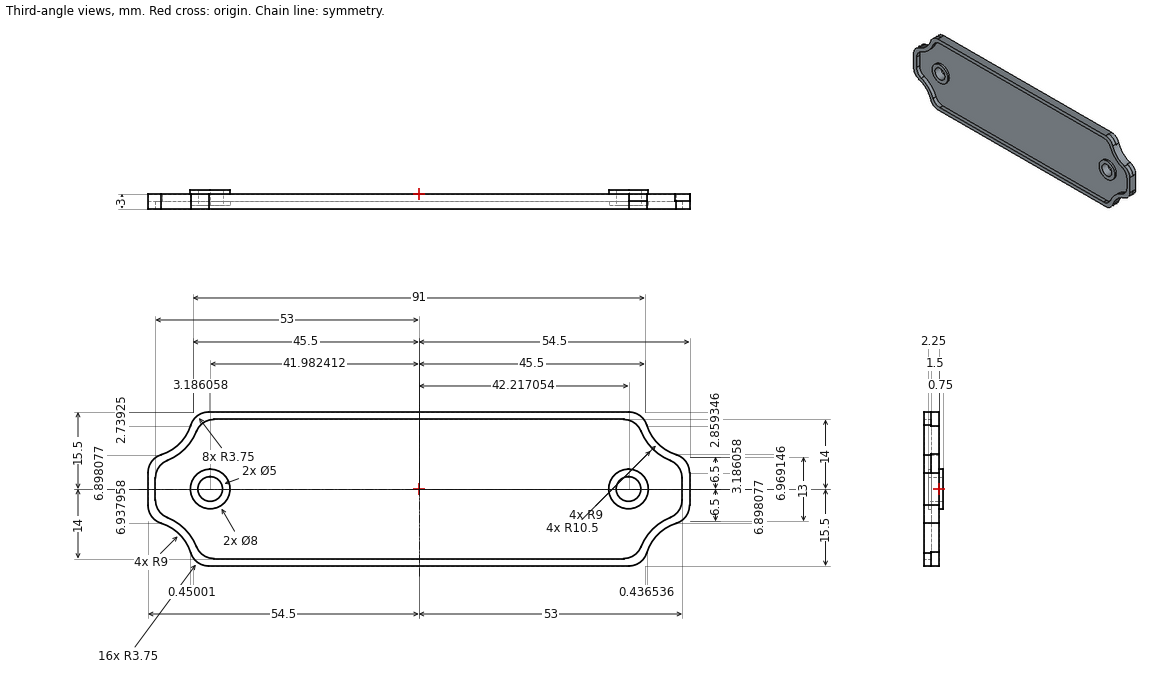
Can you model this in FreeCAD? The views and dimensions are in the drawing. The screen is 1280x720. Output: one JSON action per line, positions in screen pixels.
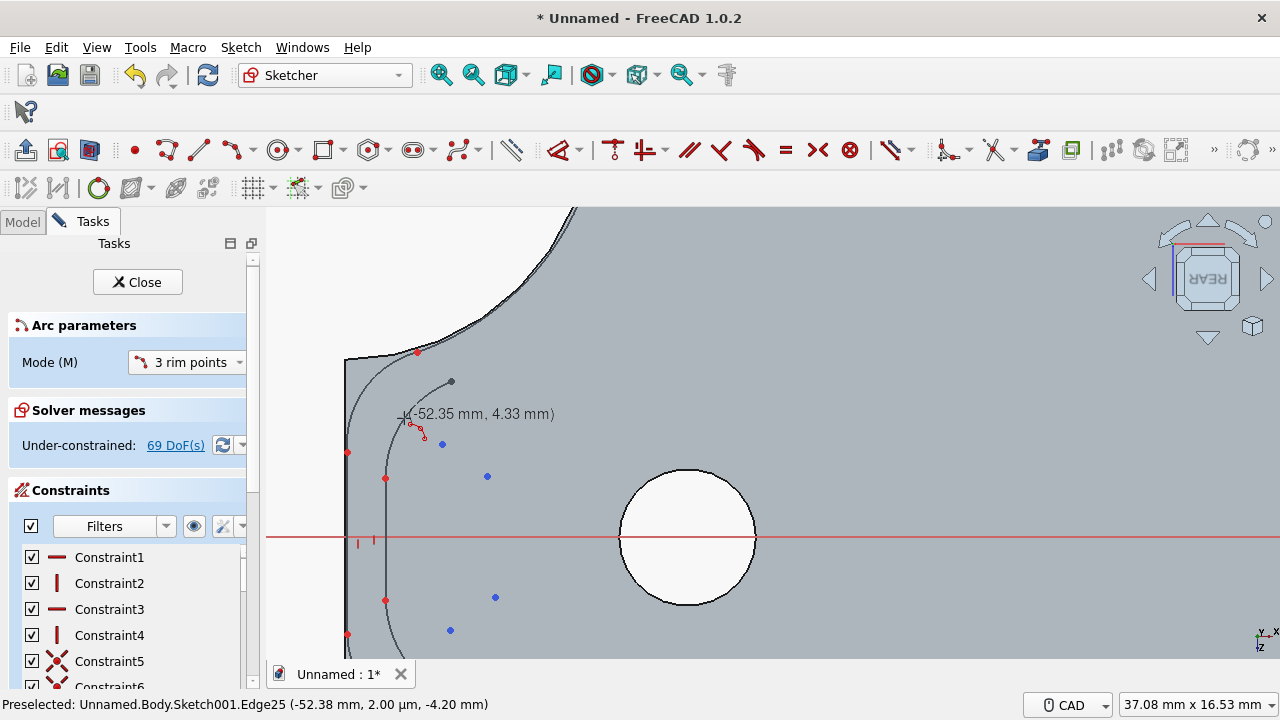
{"action": "left_click", "coordinate": [452, 382]}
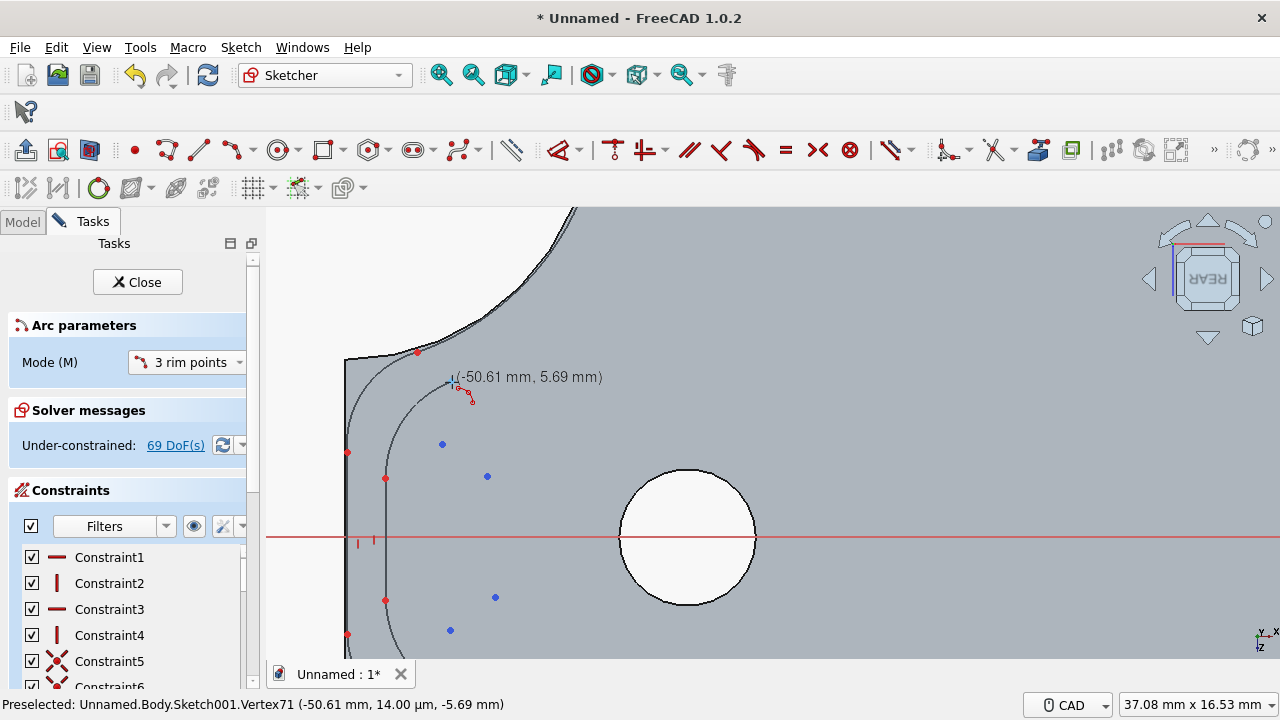
{"action": "scroll", "coordinate": [418, 407], "scroll_direction": "down", "scroll_amount": 8}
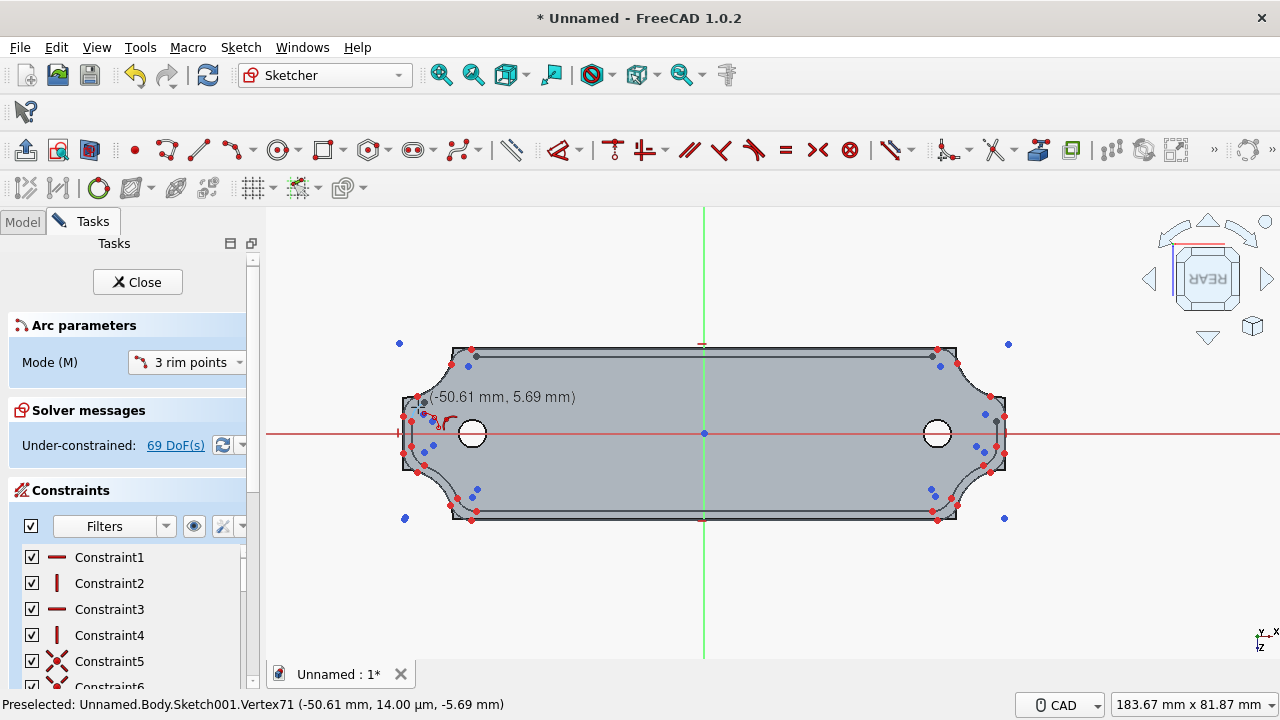
{"action": "scroll", "coordinate": [457, 369], "scroll_direction": "up", "scroll_amount": 4}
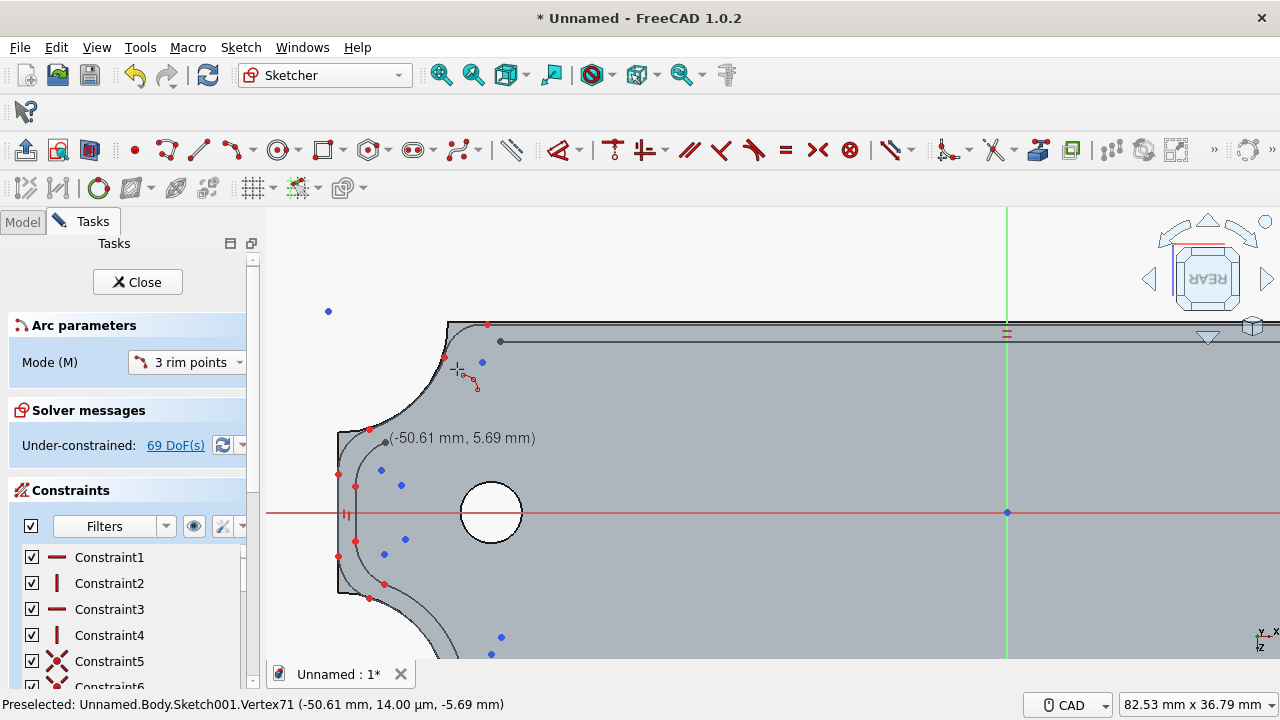
{"action": "left_click", "coordinate": [457, 370]}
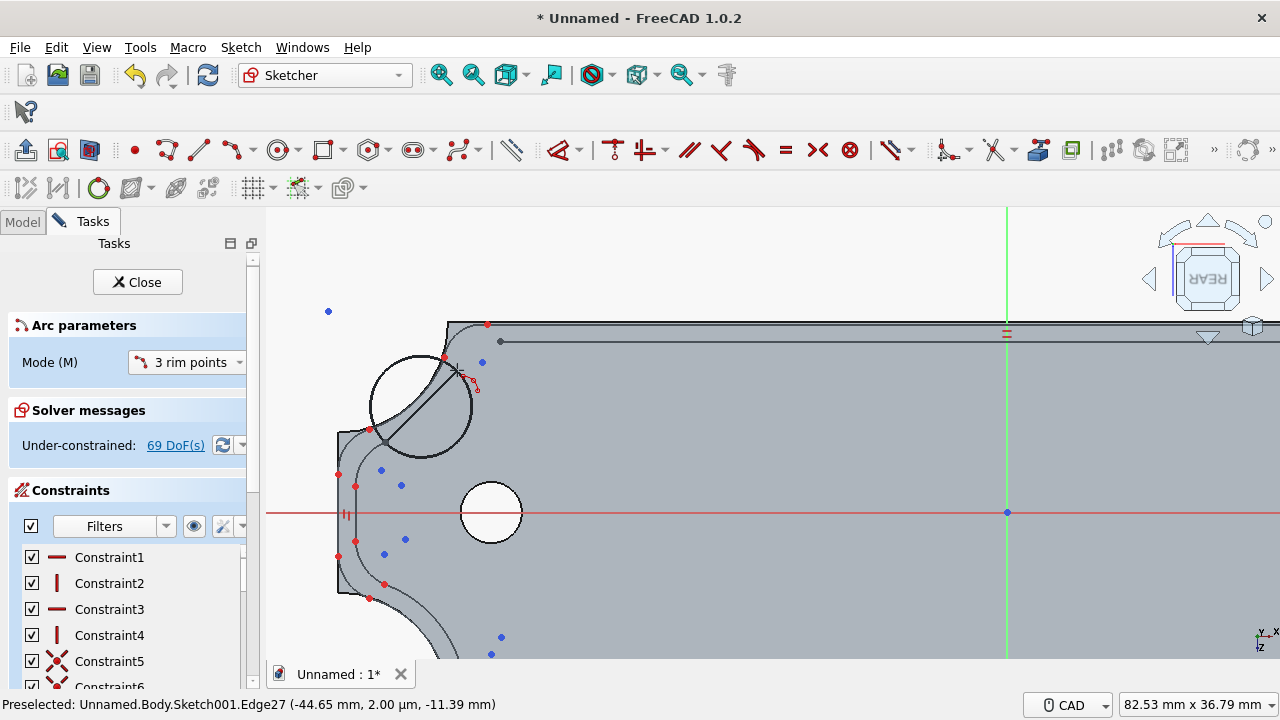
{"action": "scroll", "coordinate": [429, 413], "scroll_direction": "up", "scroll_amount": 3}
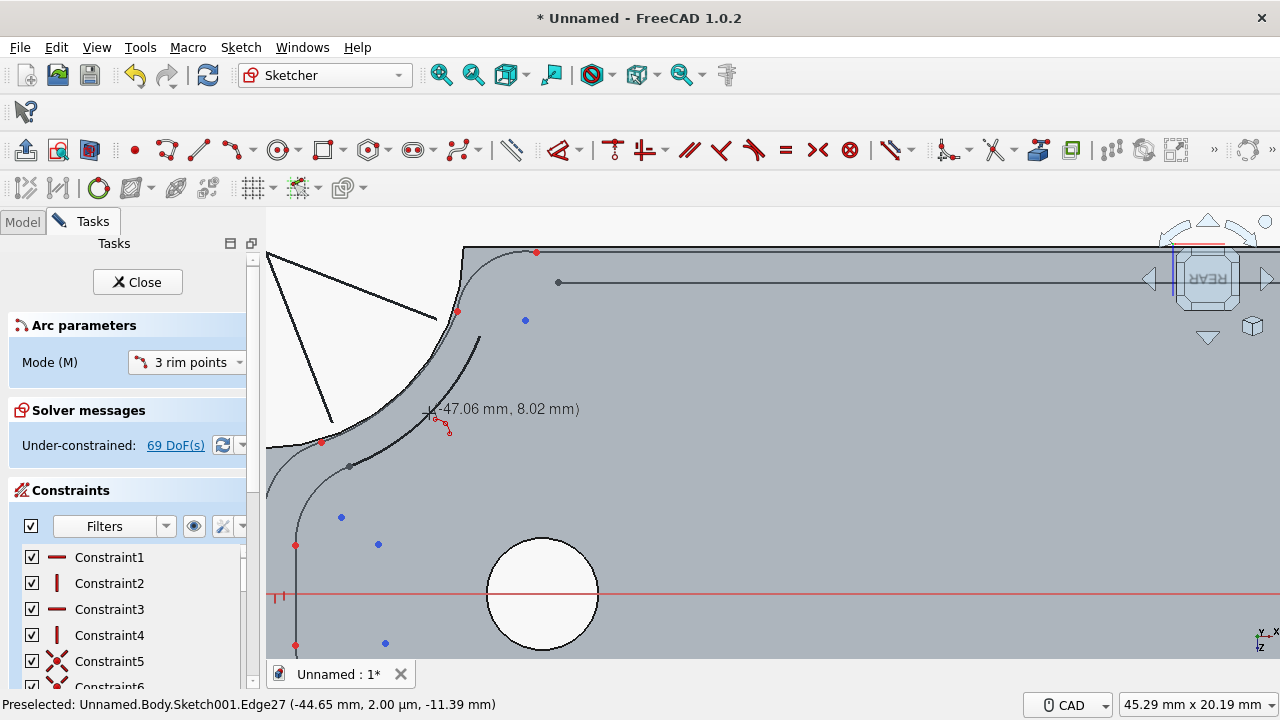
{"action": "left_click", "coordinate": [428, 413]}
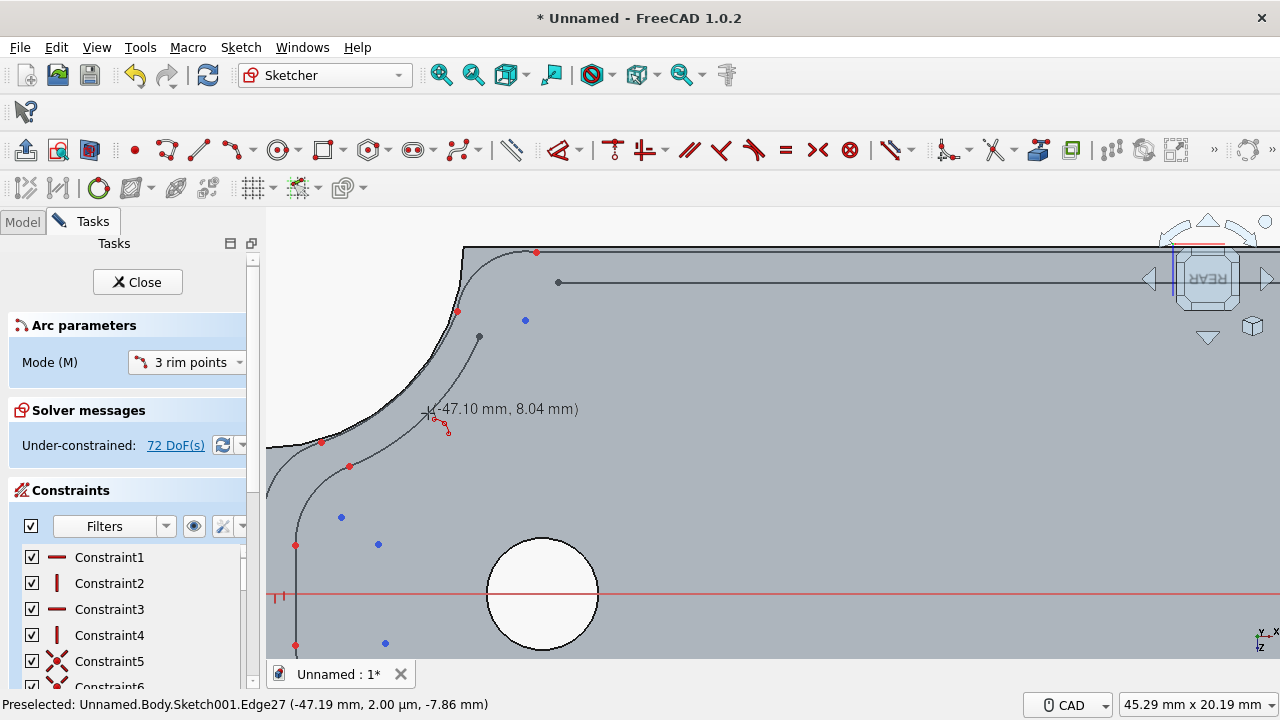
{"action": "left_click", "coordinate": [480, 336]}
{"action": "left_click", "coordinate": [558, 283]}
{"action": "left_click", "coordinate": [512, 295]}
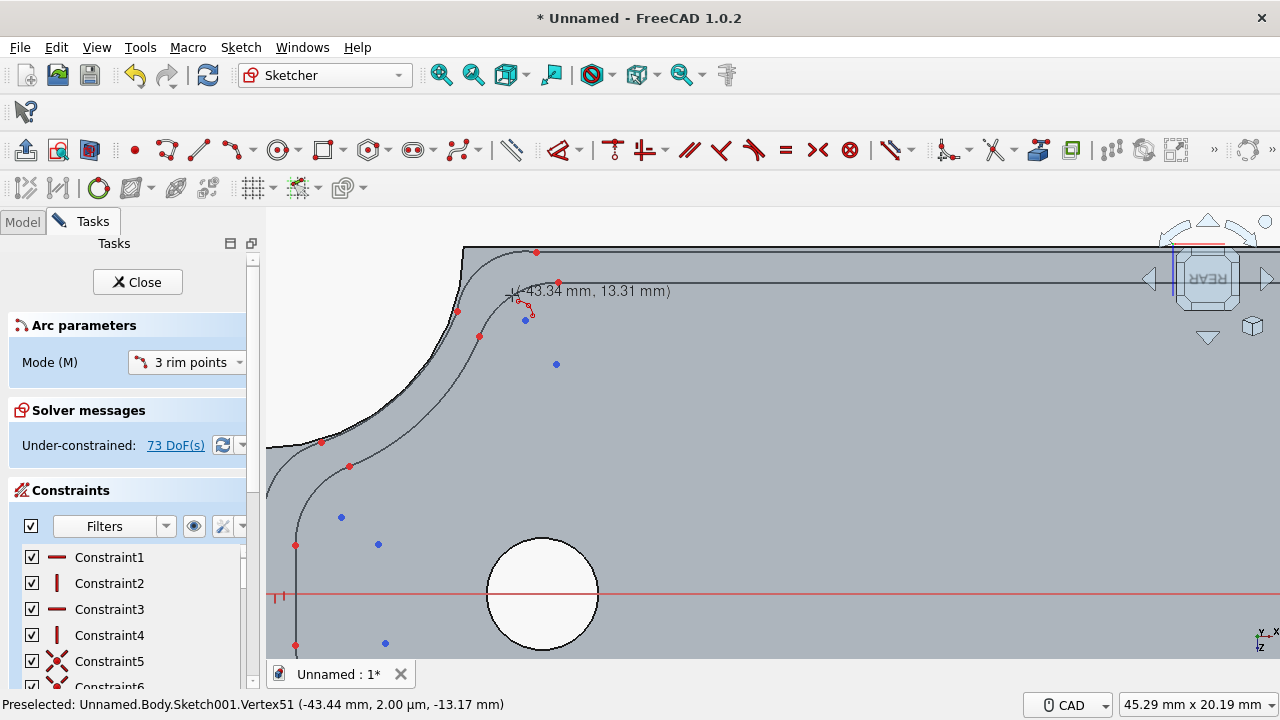
{"action": "scroll", "coordinate": [450, 380], "scroll_direction": "down", "scroll_amount": 7}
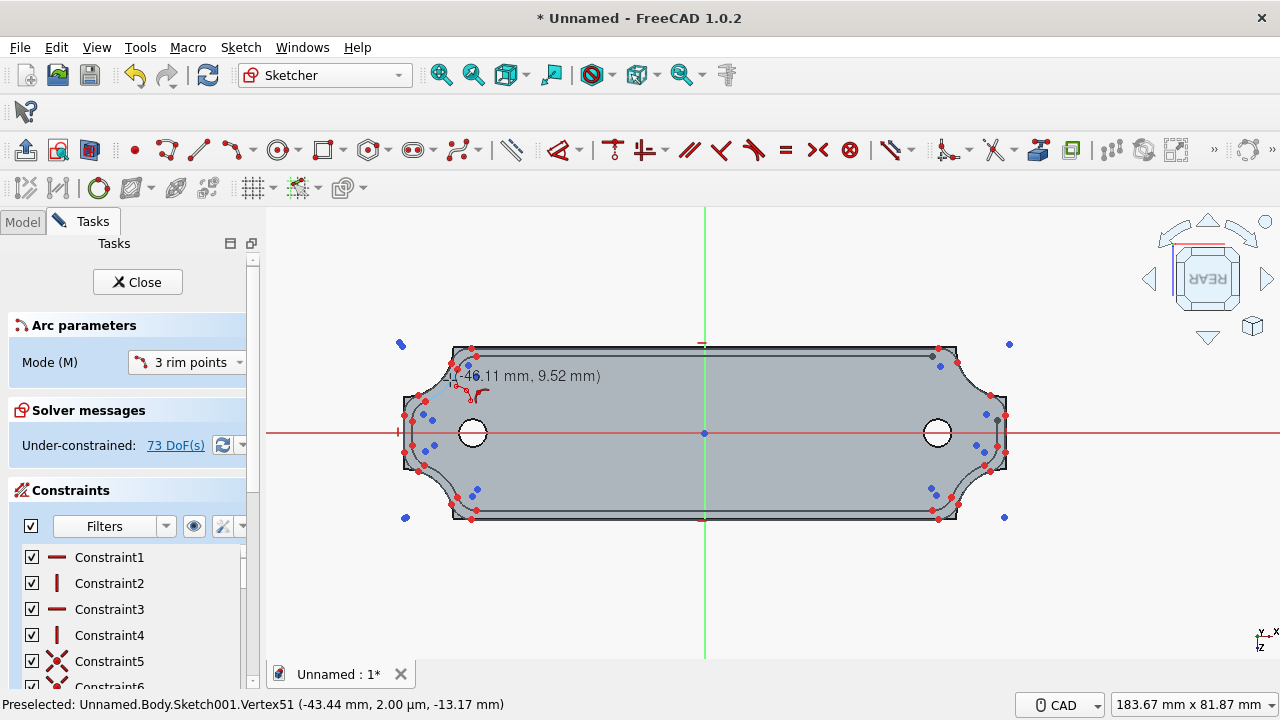
{"action": "scroll", "coordinate": [932, 356], "scroll_direction": "up", "scroll_amount": 4}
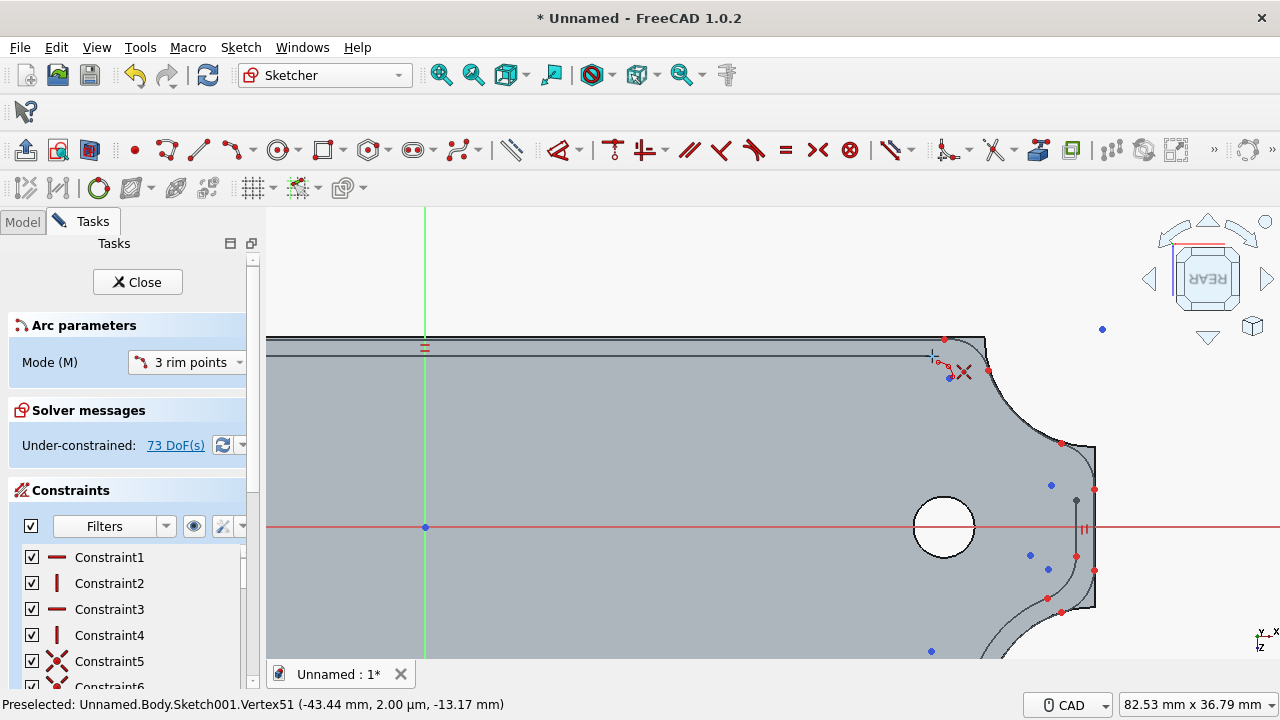
{"action": "left_click", "coordinate": [932, 356]}
{"action": "left_click", "coordinate": [975, 384]}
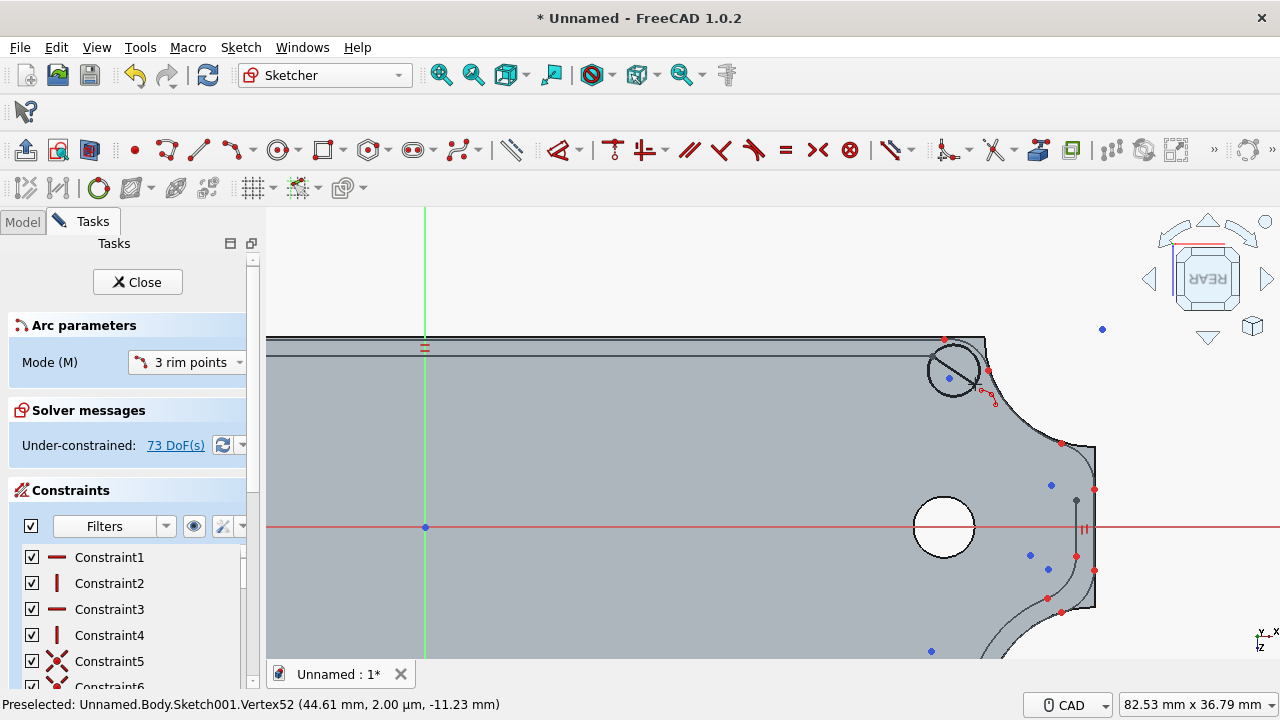
{"action": "scroll", "coordinate": [958, 363], "scroll_direction": "up", "scroll_amount": 4}